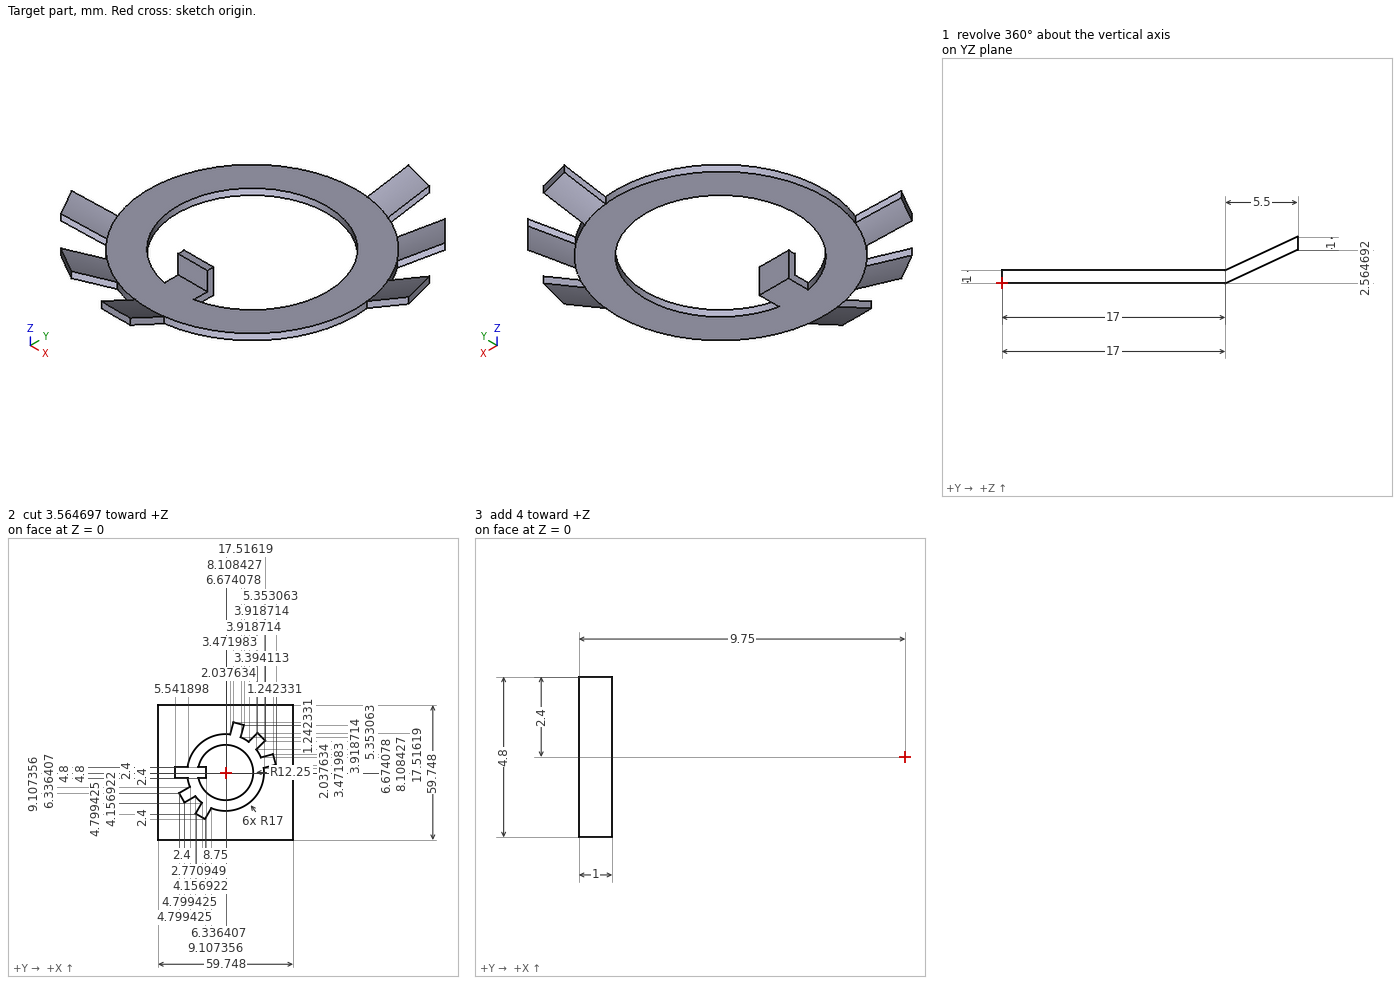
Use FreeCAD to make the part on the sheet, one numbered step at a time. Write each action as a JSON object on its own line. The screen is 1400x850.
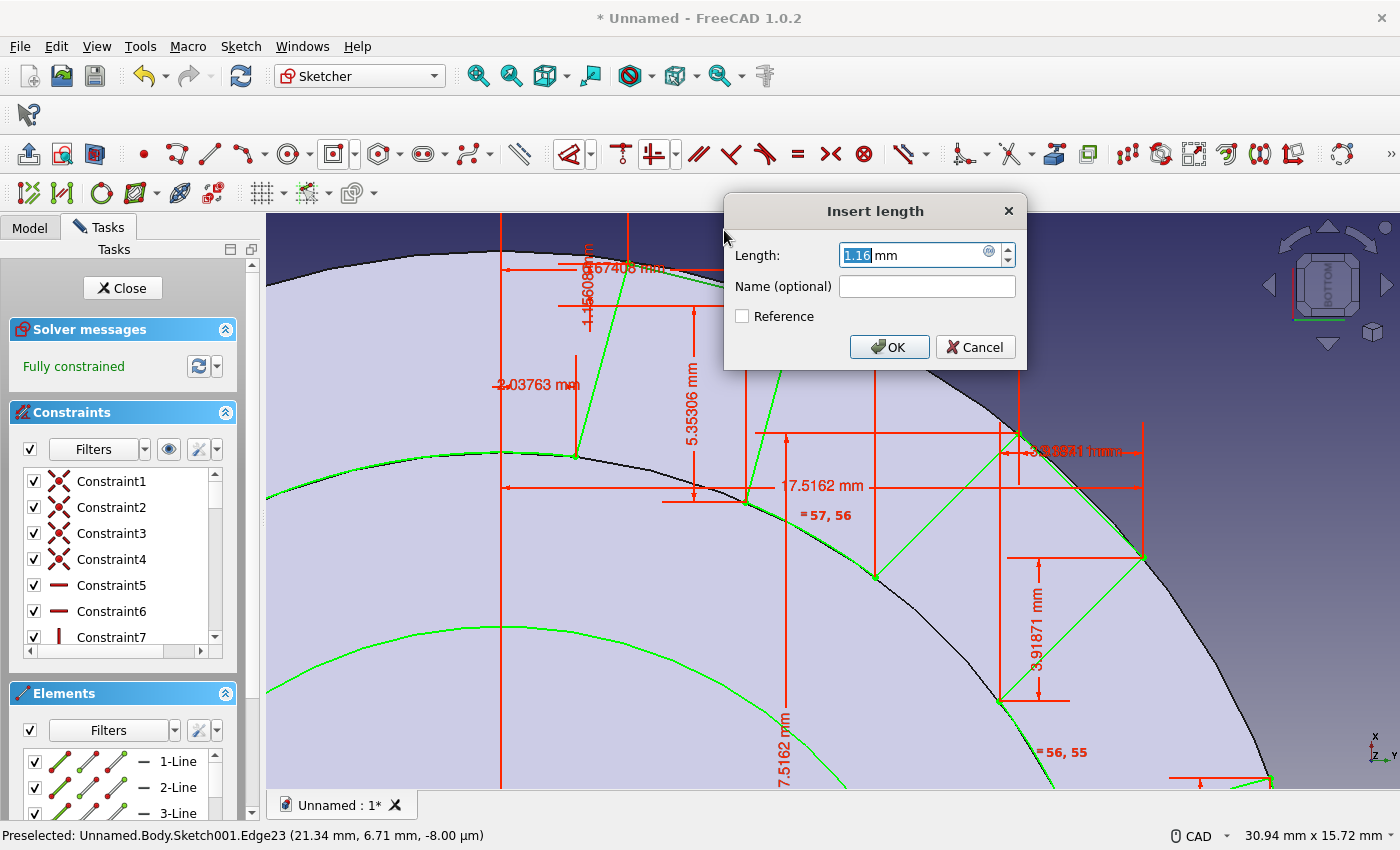
{"action": "type", "text": "1.242331"}
{"action": "key", "text": "Return"}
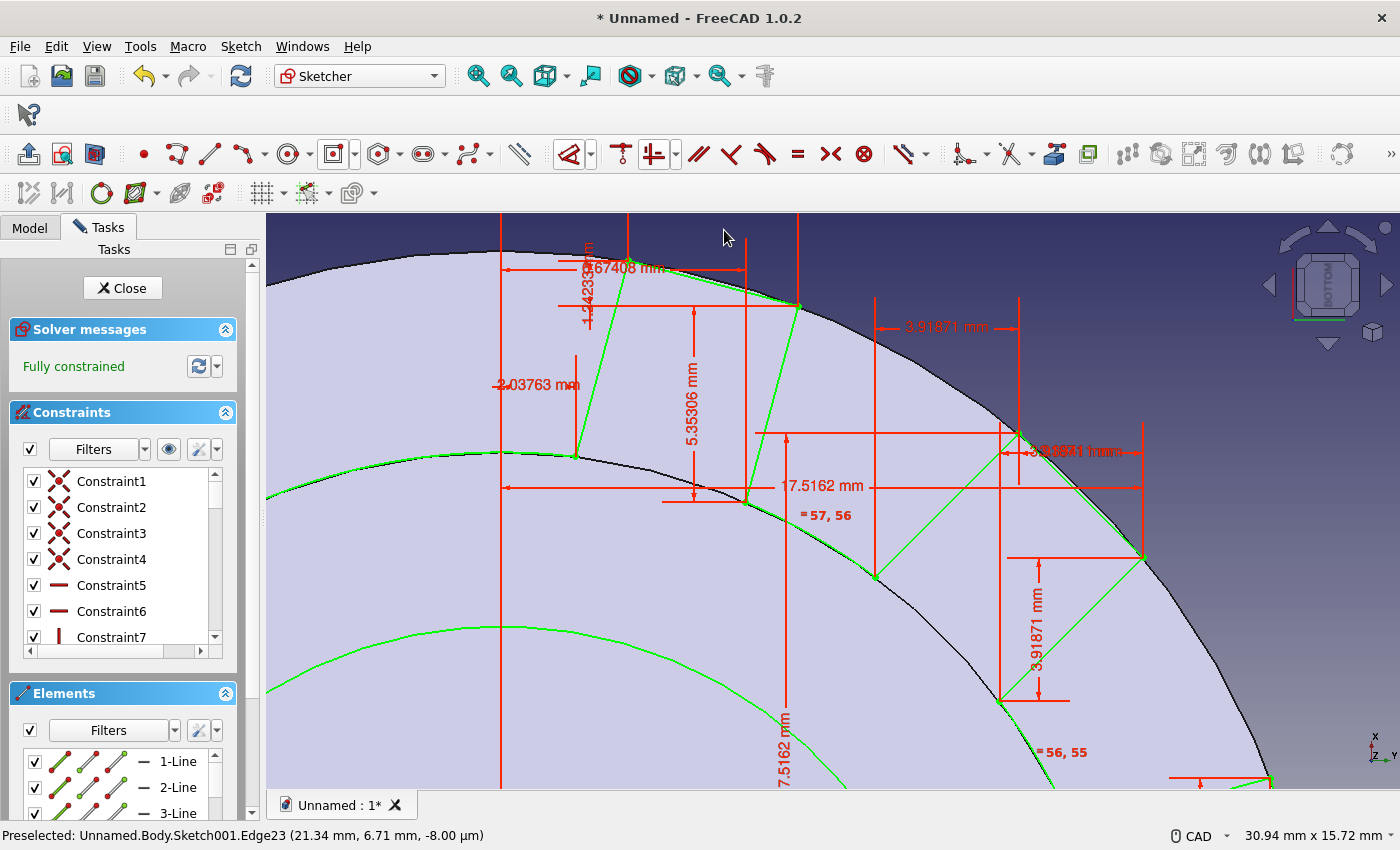
{"action": "left_click", "coordinate": [123, 288]}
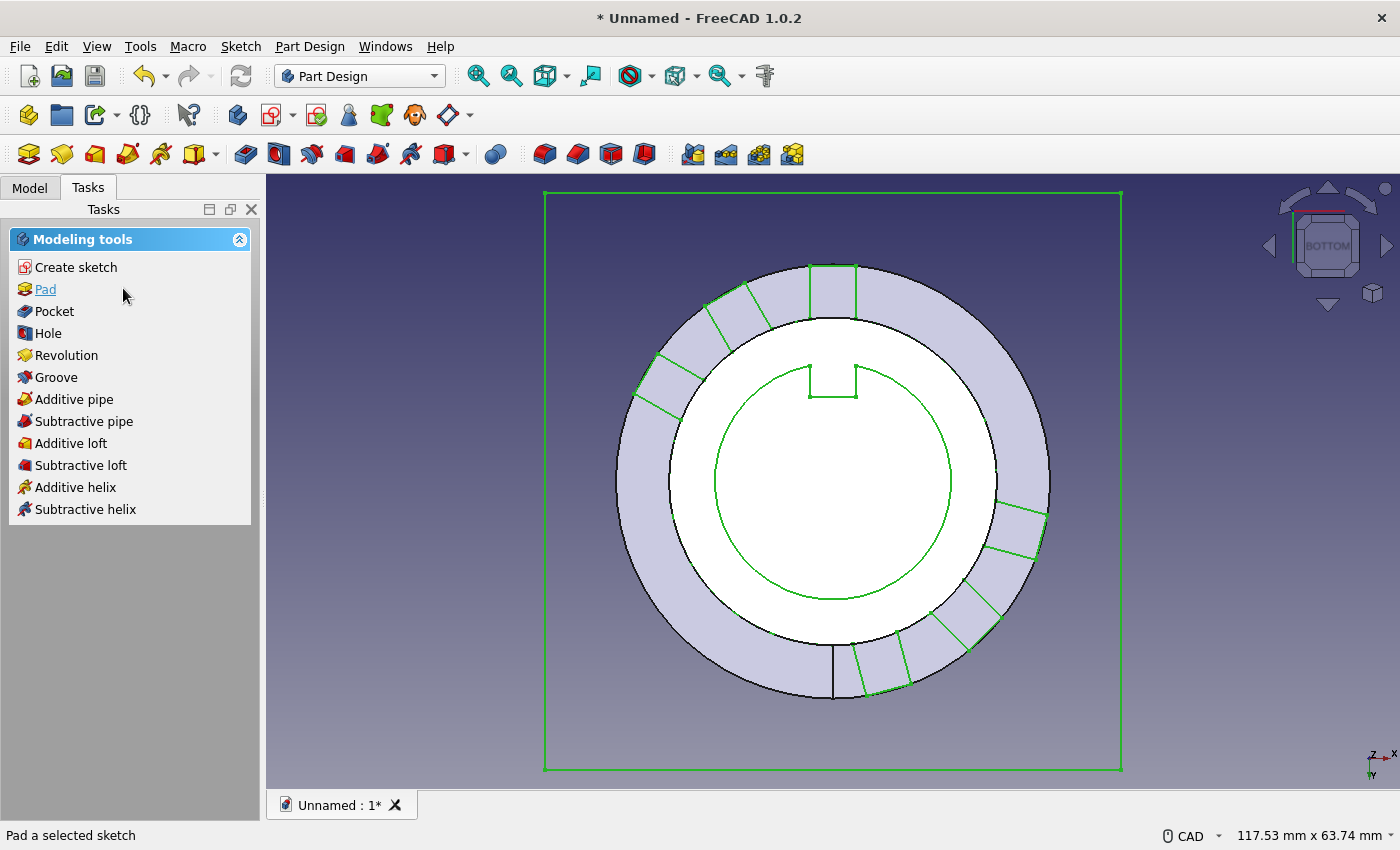
{"action": "left_click", "coordinate": [246, 154]}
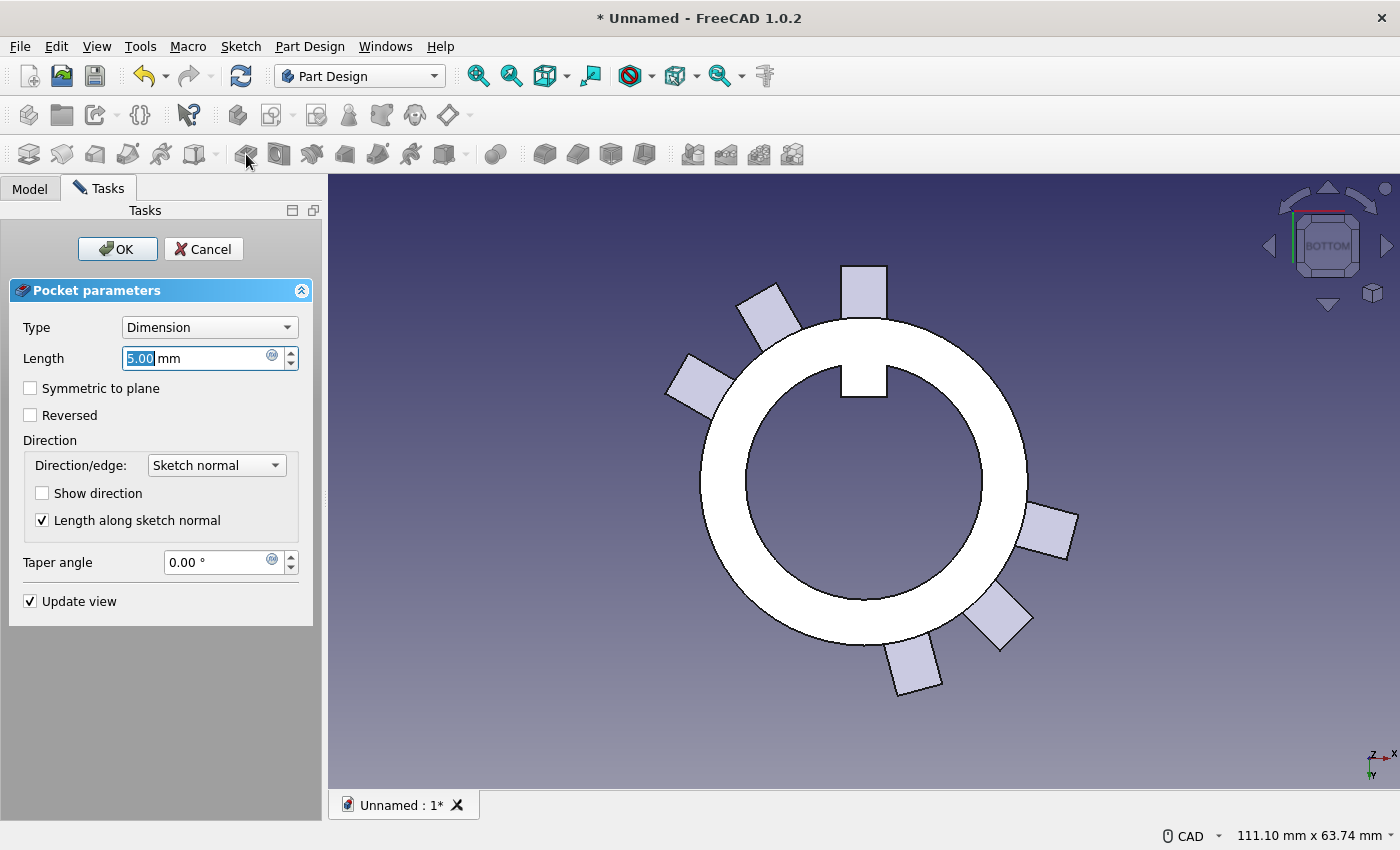
{"action": "type", "text": "3.564697"}
{"action": "key", "text": "Tab"}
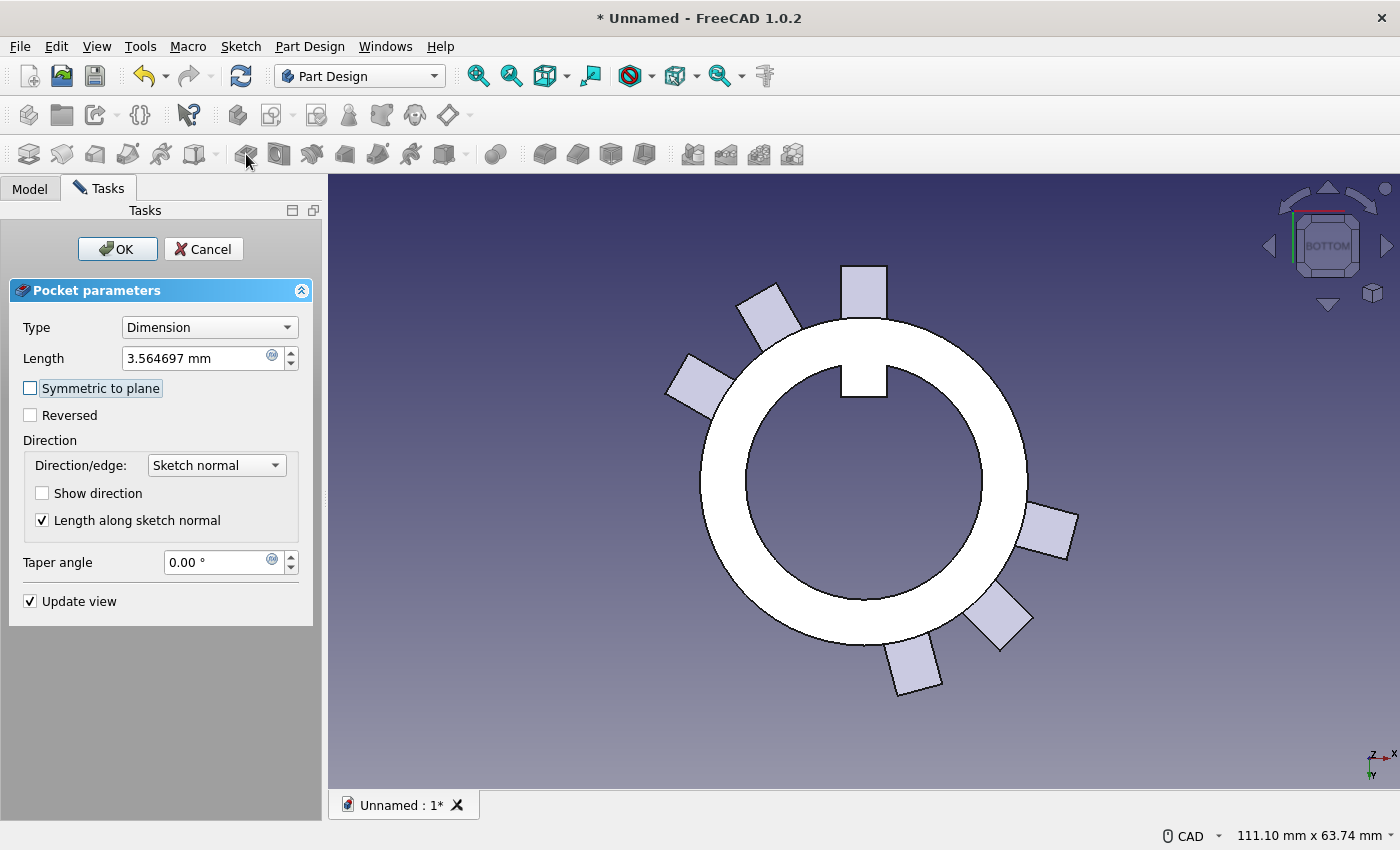
{"action": "left_click", "coordinate": [118, 249]}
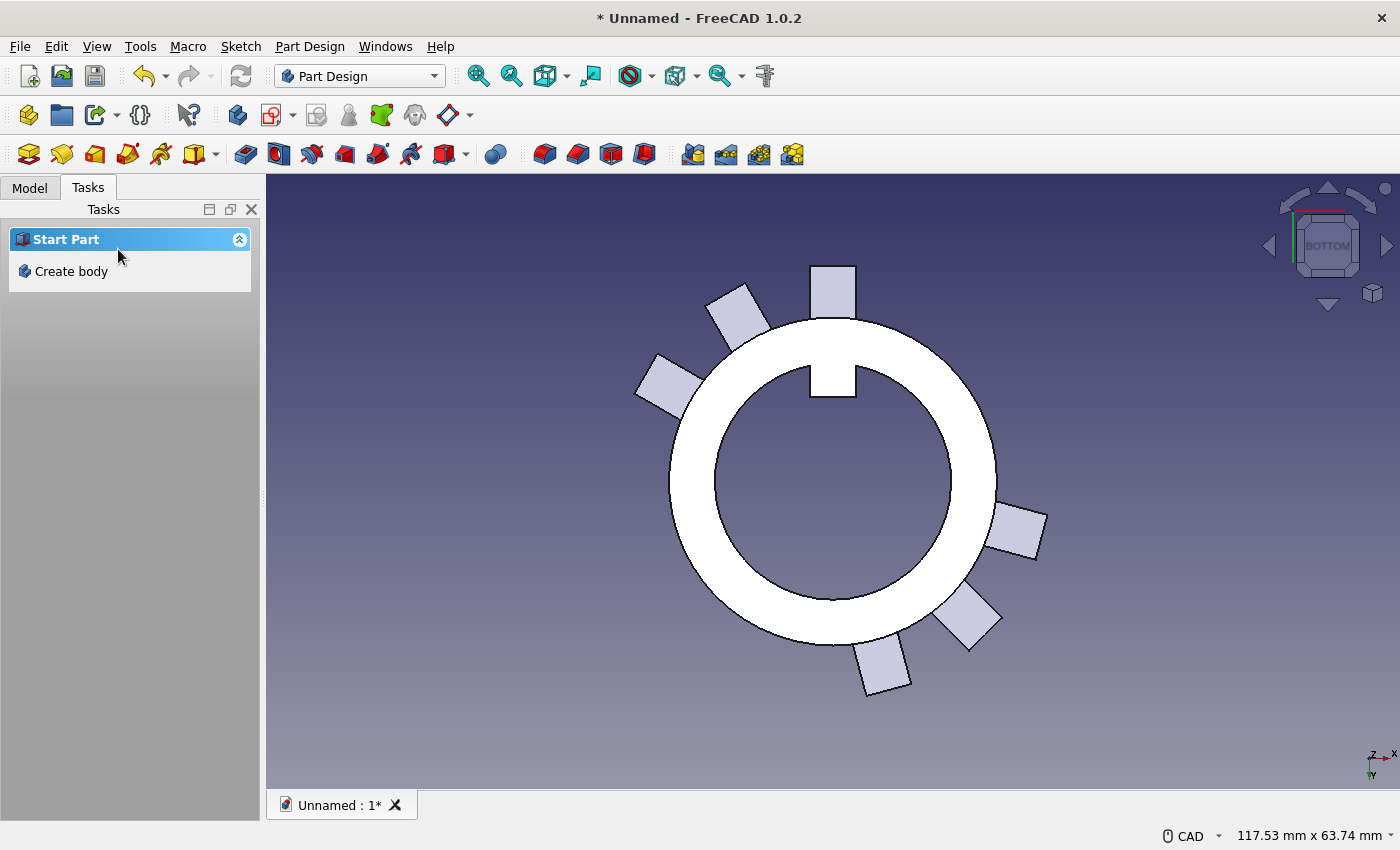
{"action": "left_click", "coordinate": [833, 340]}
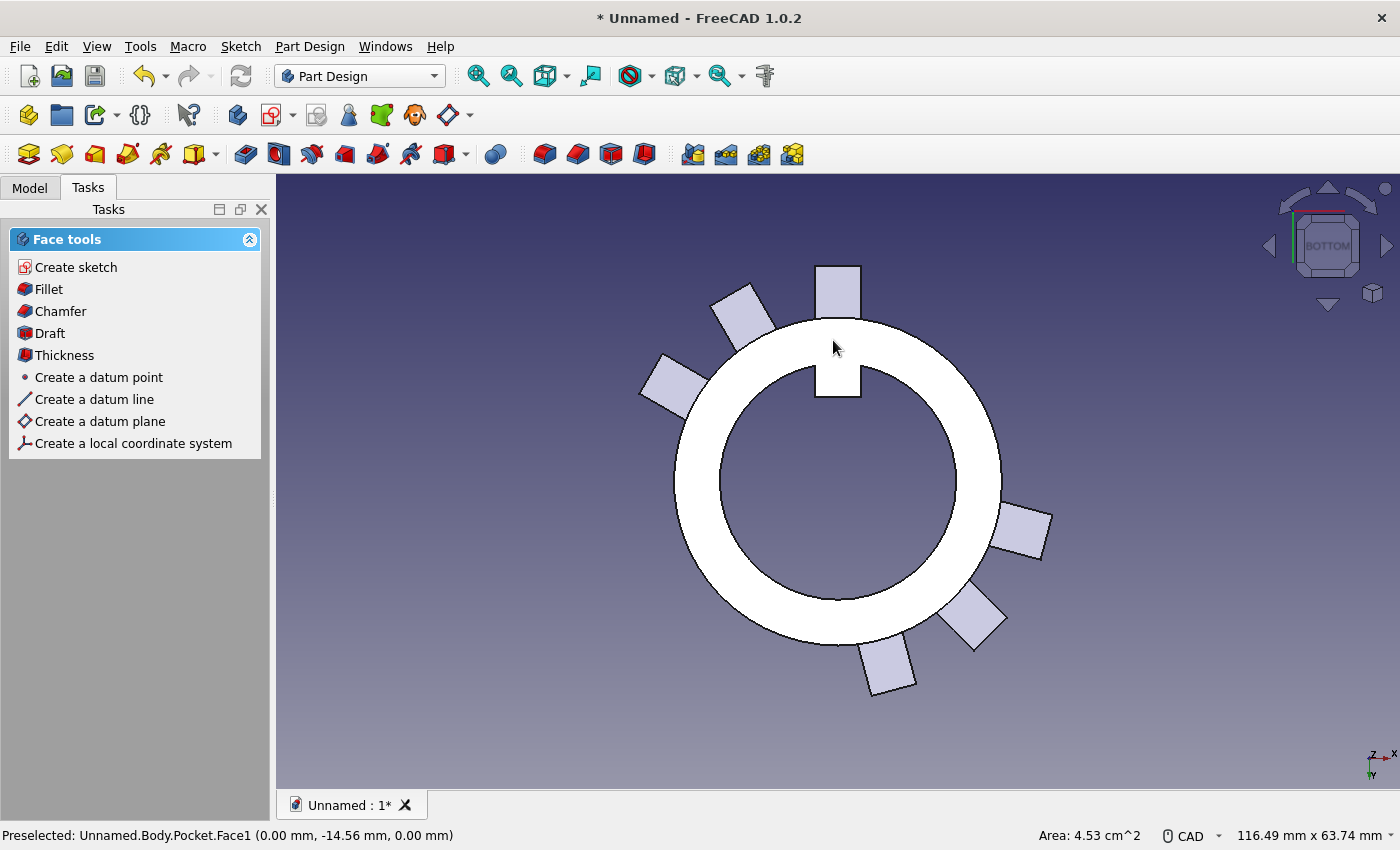
{"action": "left_click", "coordinate": [270, 116]}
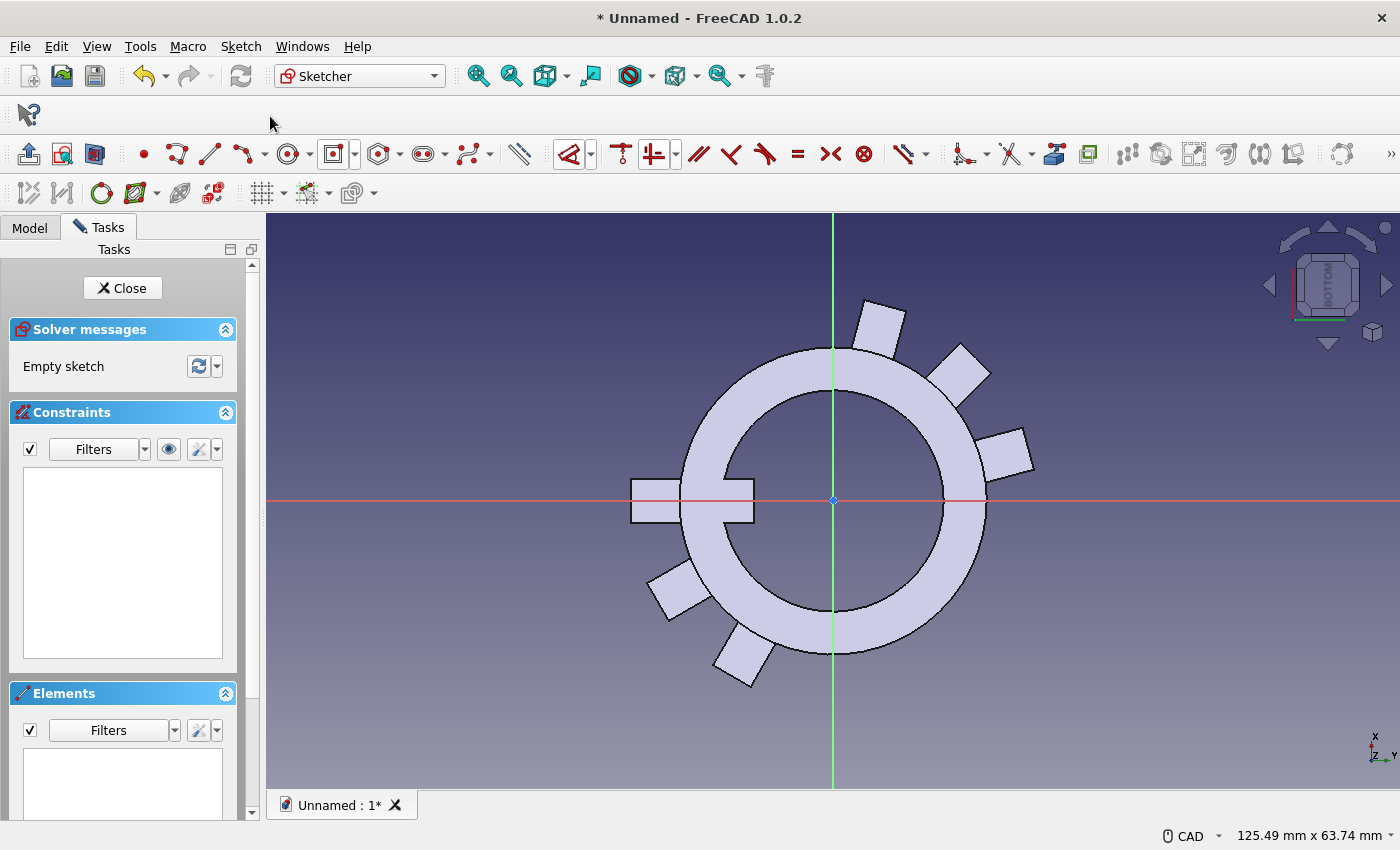
{"action": "scroll", "coordinate": [793, 501], "scroll_direction": "up", "scroll_amount": 10}